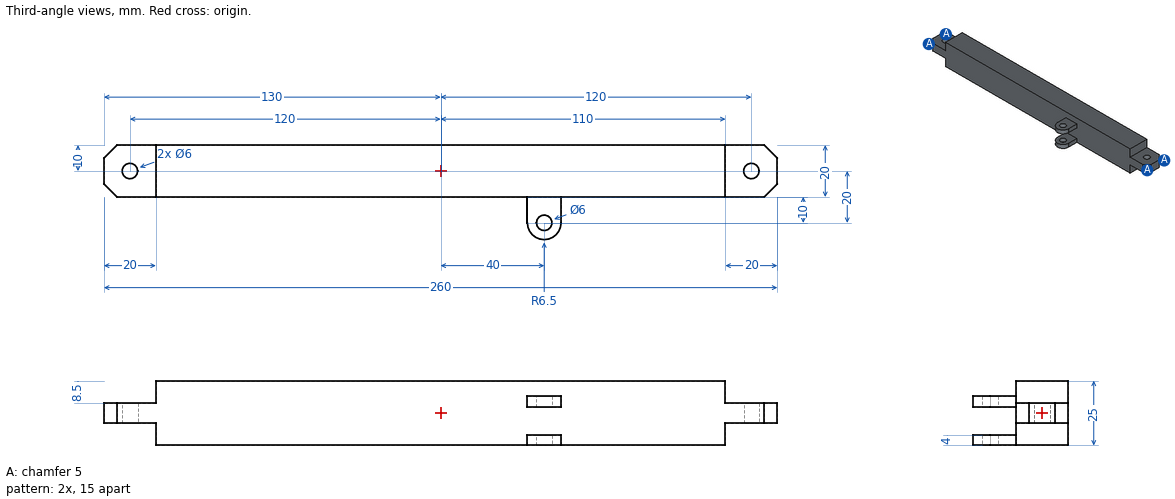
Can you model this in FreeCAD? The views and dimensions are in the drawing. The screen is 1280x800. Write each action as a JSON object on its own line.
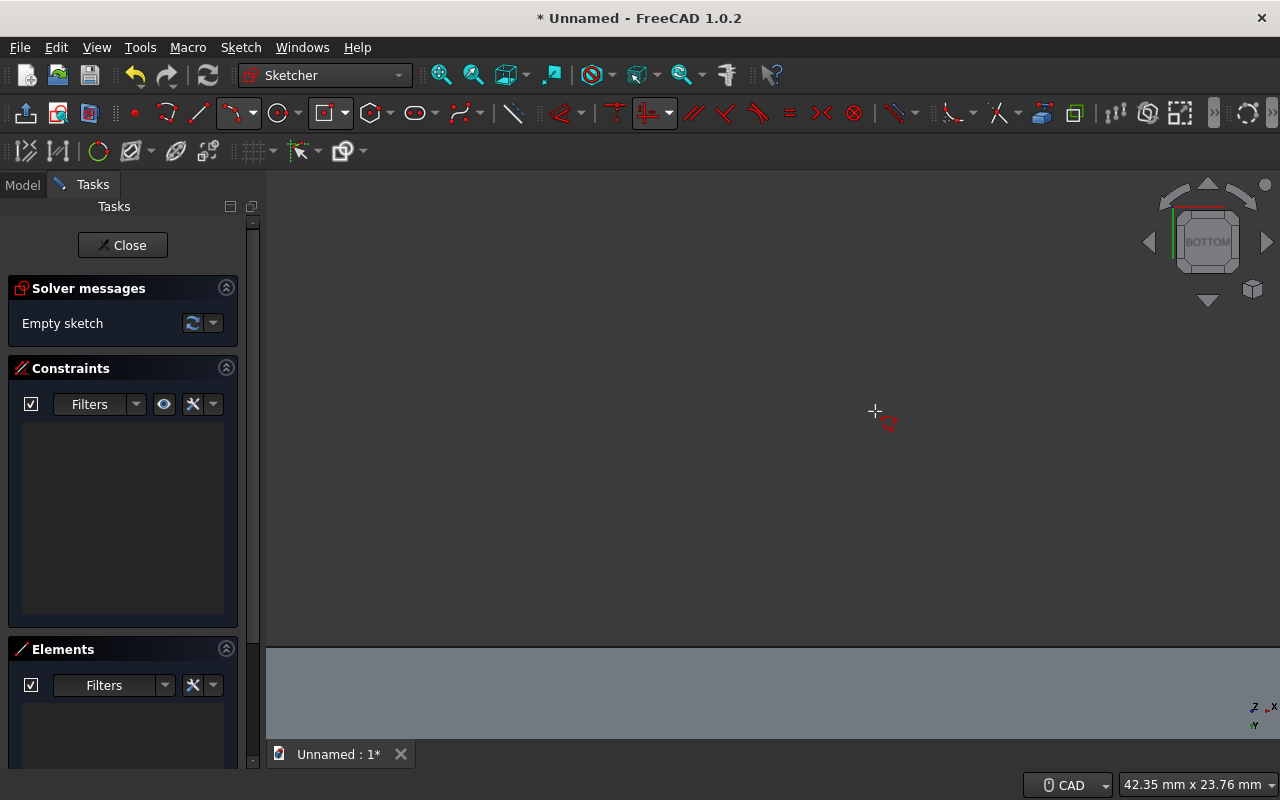
{"action": "left_click", "coordinate": [547, 407]}
{"action": "left_click", "coordinate": [547, 647]}
{"action": "left_click", "coordinate": [858, 647]}
{"action": "left_click", "coordinate": [858, 407]}
{"action": "right_click", "coordinate": [858, 407]}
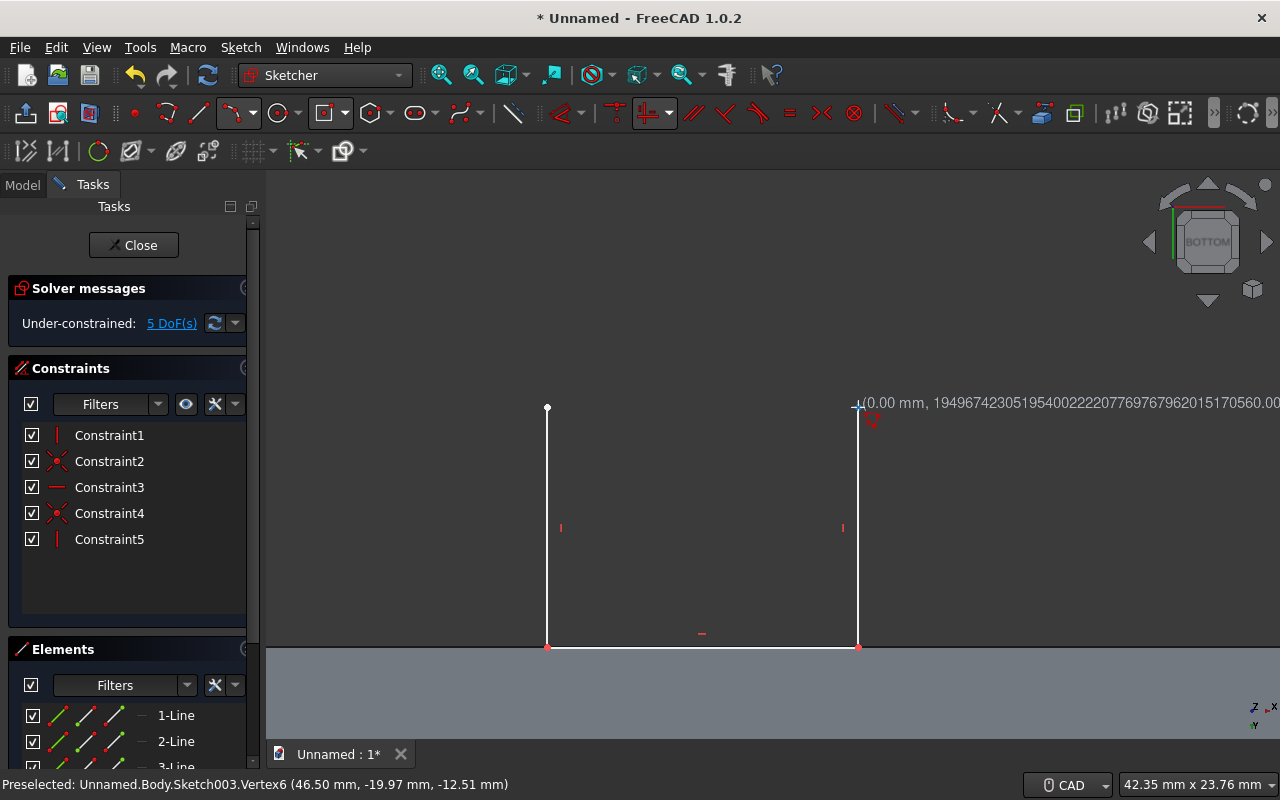
{"action": "left_click", "coordinate": [232, 114]}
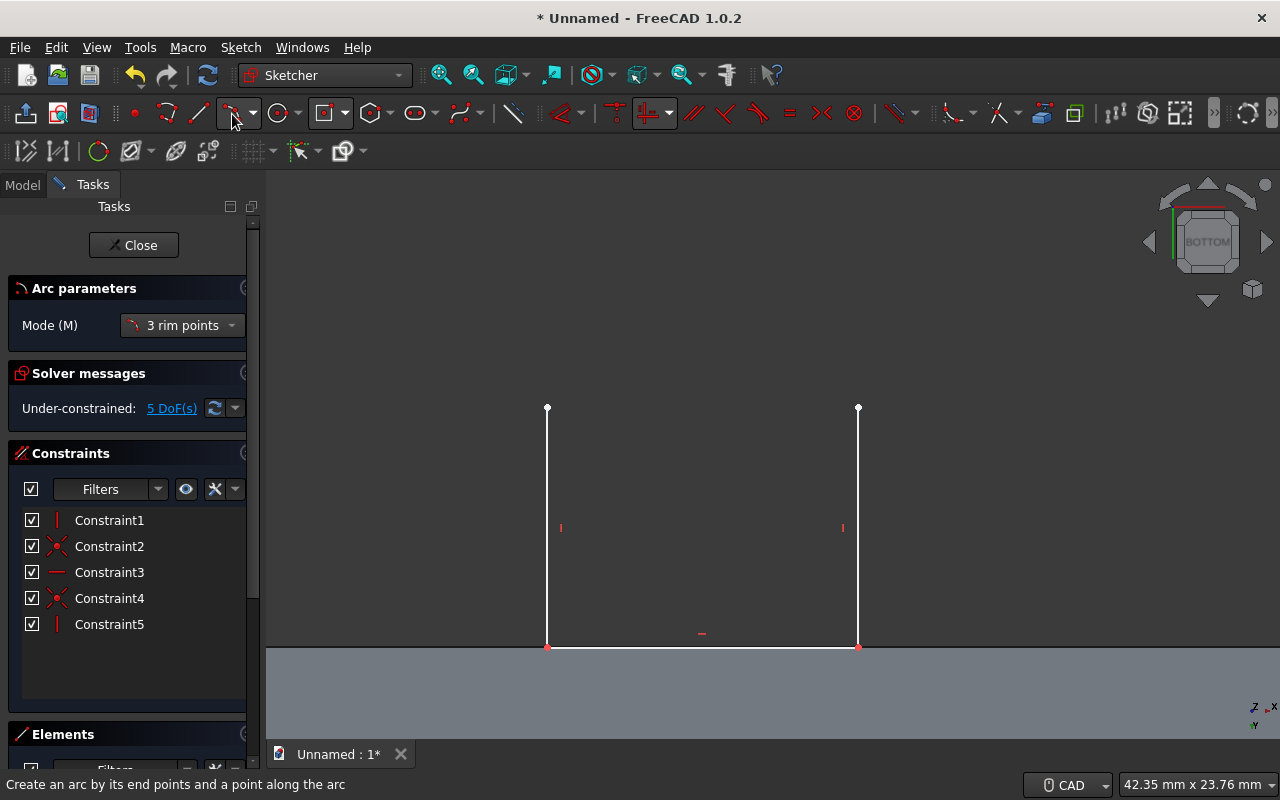
{"action": "left_click", "coordinate": [858, 408]}
{"action": "left_click", "coordinate": [547, 408]}
{"action": "left_click", "coordinate": [702, 252]}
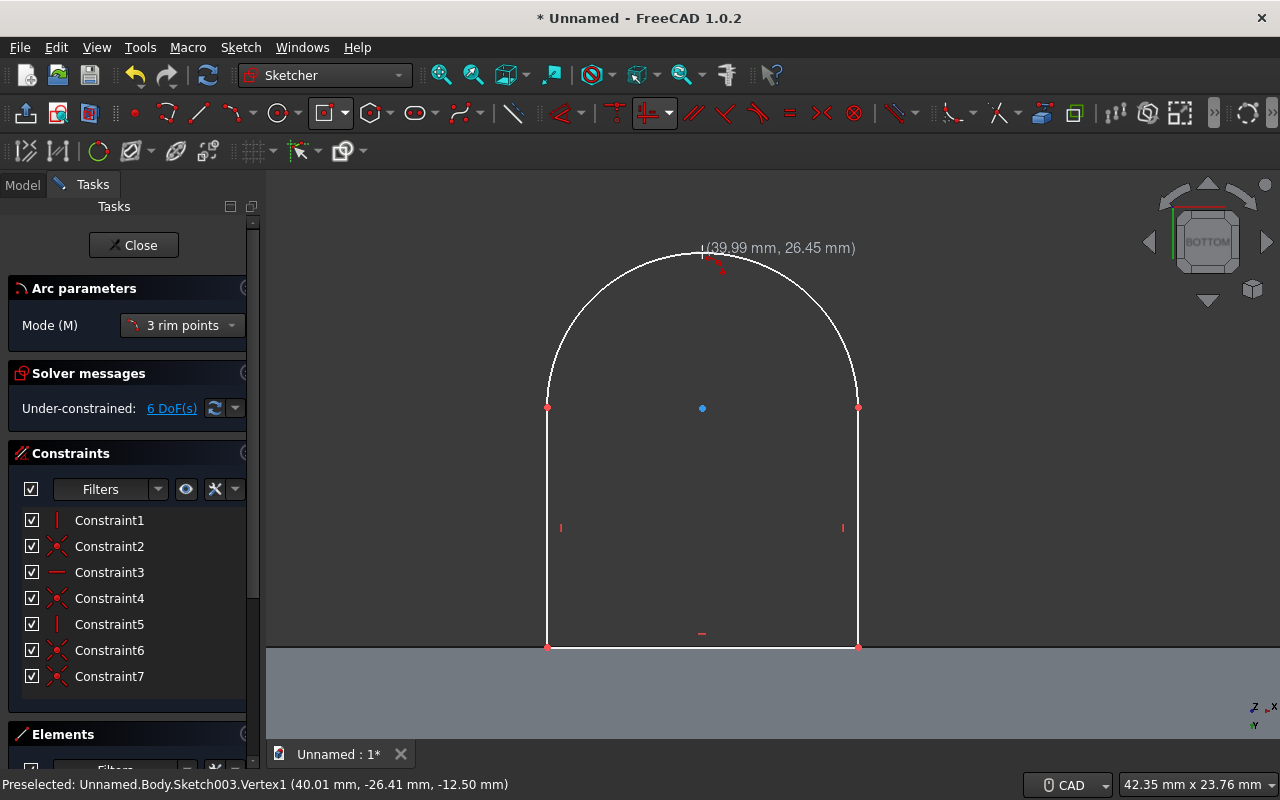
{"action": "key", "text": "g c"}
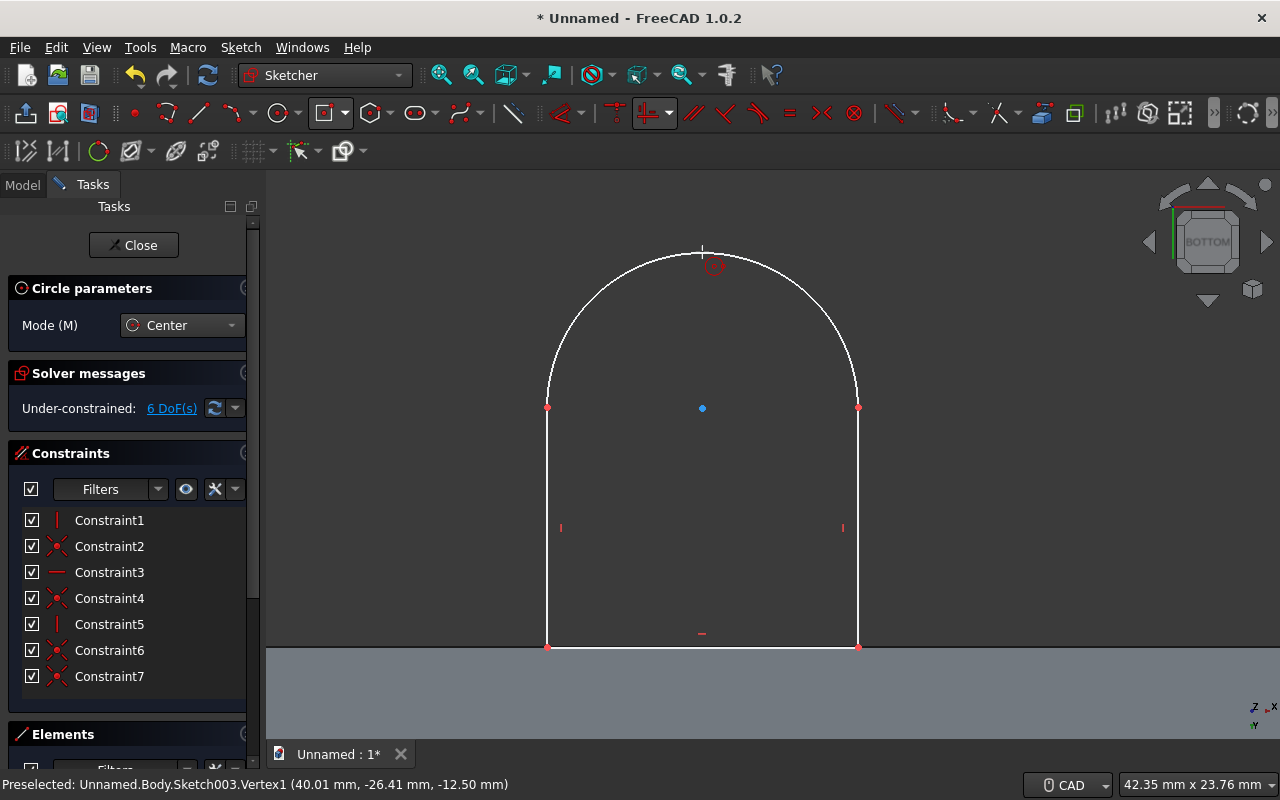
{"action": "left_click", "coordinate": [702, 407]}
{"action": "mouse_move", "coordinate": [753, 357]}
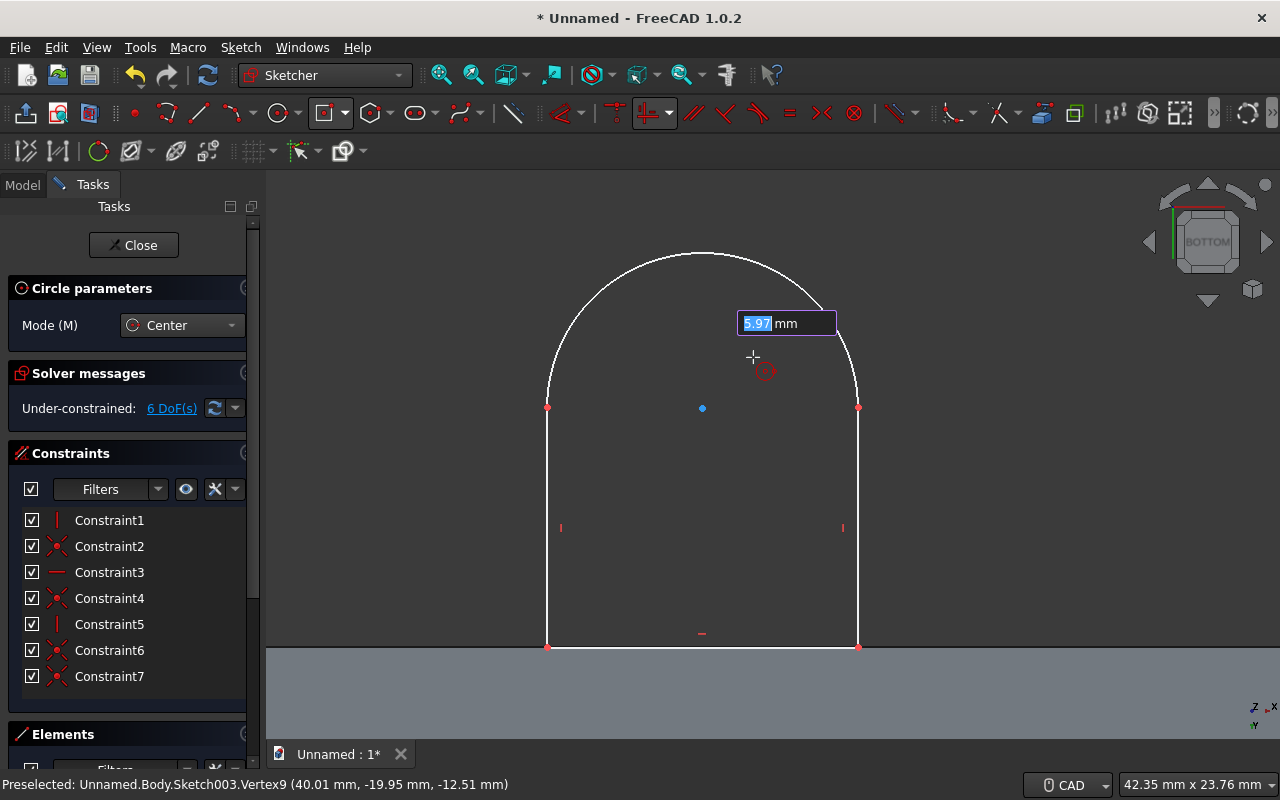
{"action": "type", "text": "6"}
{"action": "key", "text": "Return"}
{"action": "key", "text": "Escape"}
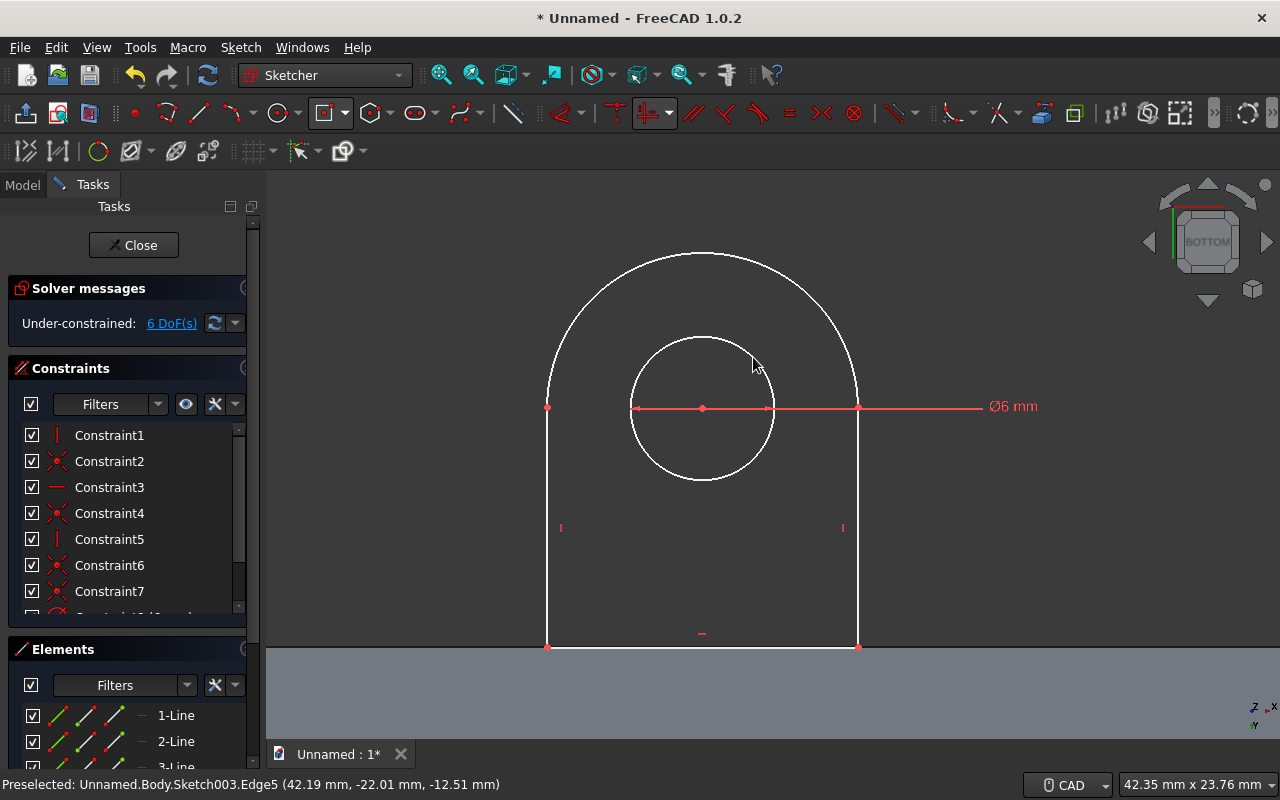
{"action": "left_click", "coordinate": [547, 480]}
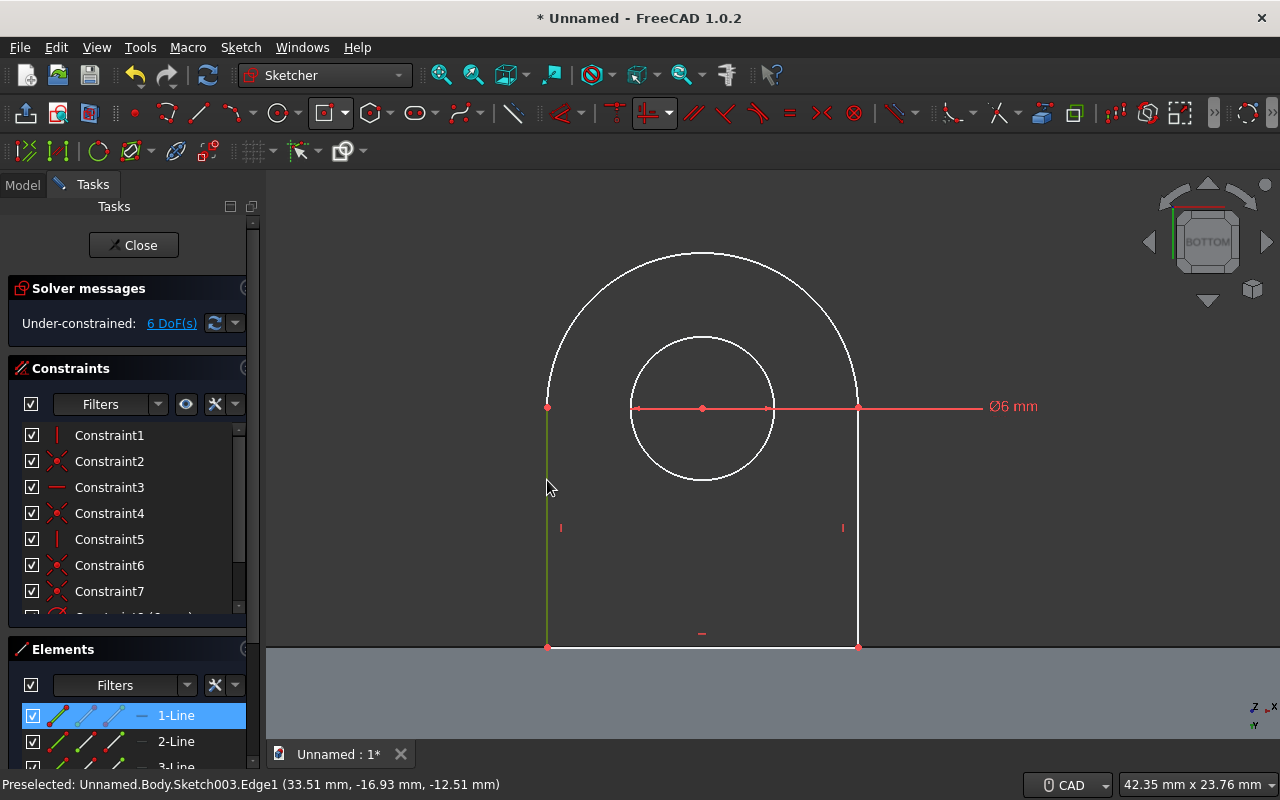
{"action": "left_click", "coordinate": [794, 283]}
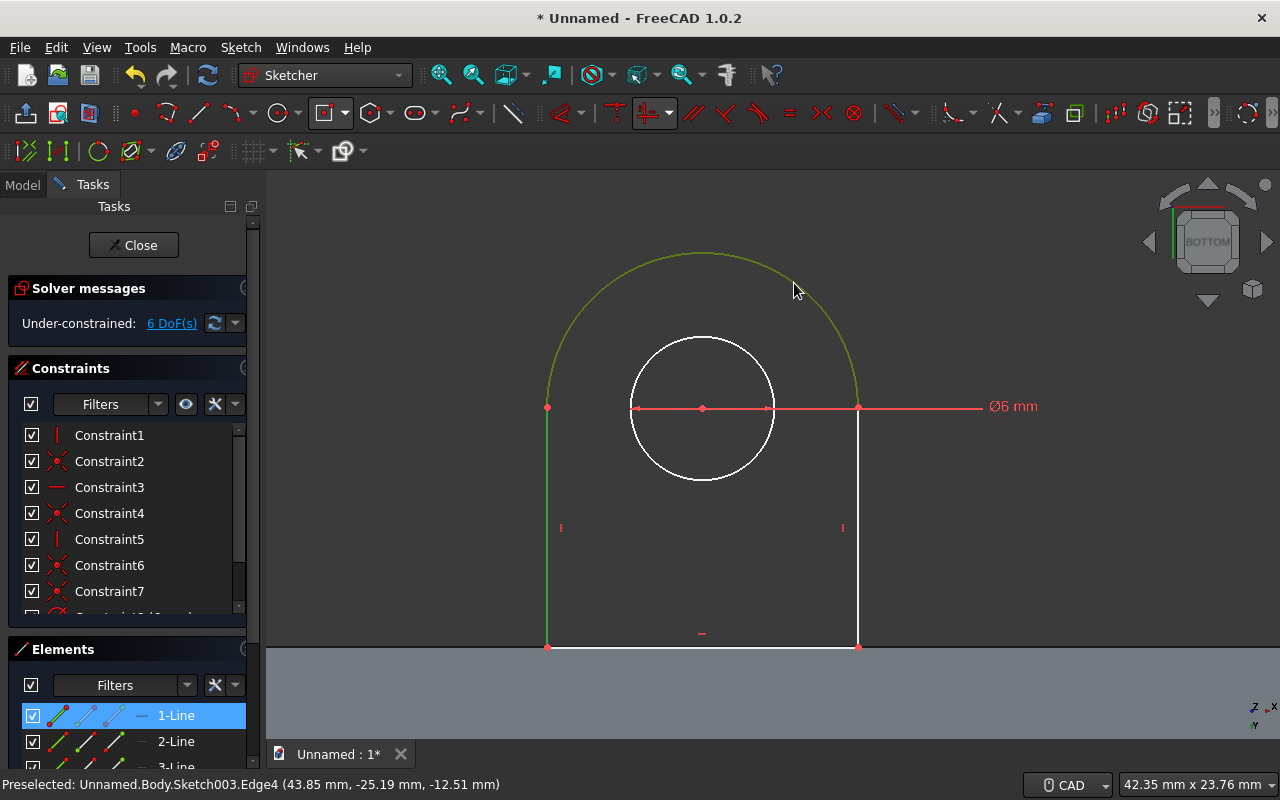
{"action": "left_click", "coordinate": [758, 114]}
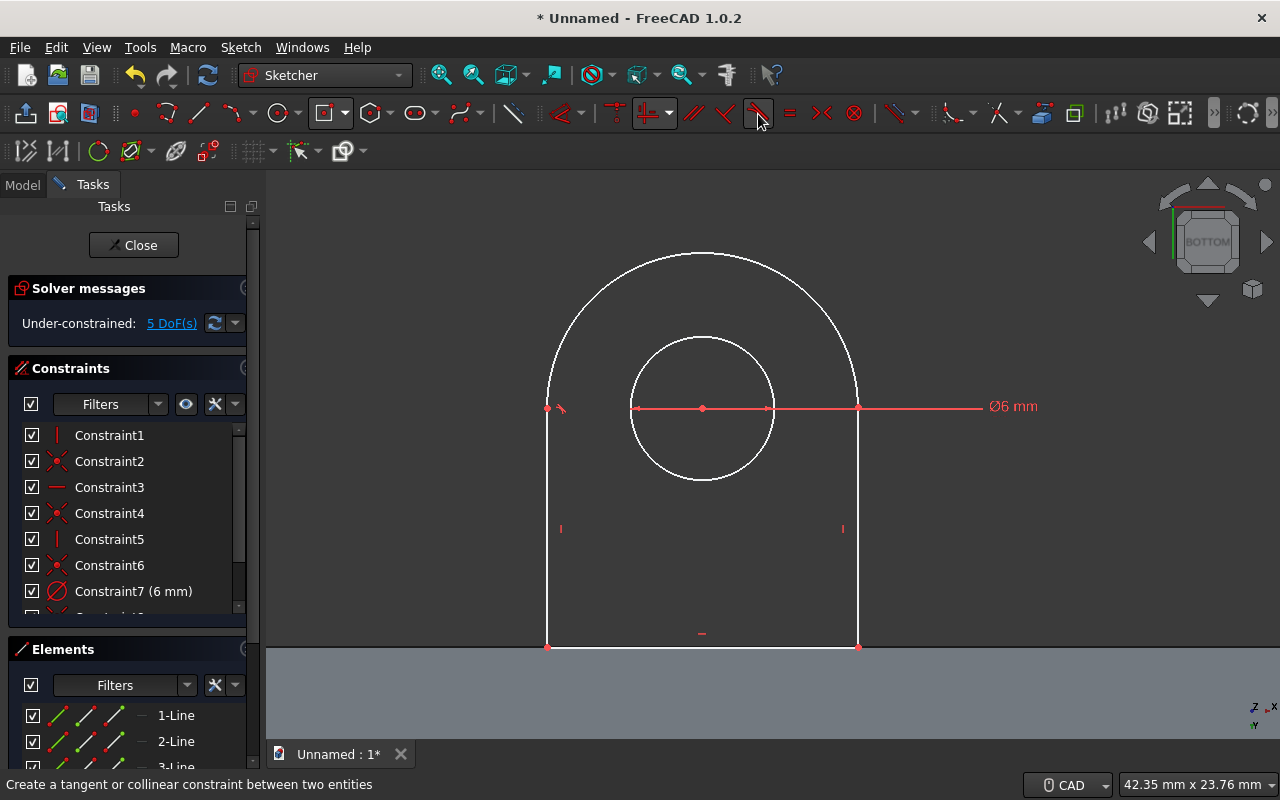
{"action": "left_click", "coordinate": [858, 576]}